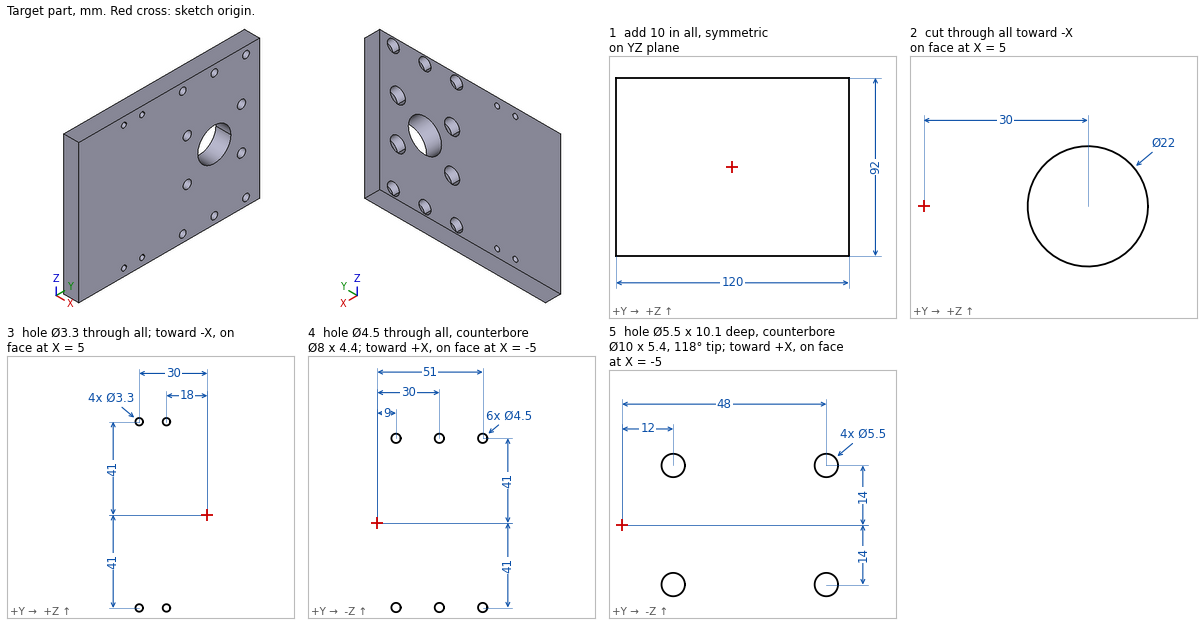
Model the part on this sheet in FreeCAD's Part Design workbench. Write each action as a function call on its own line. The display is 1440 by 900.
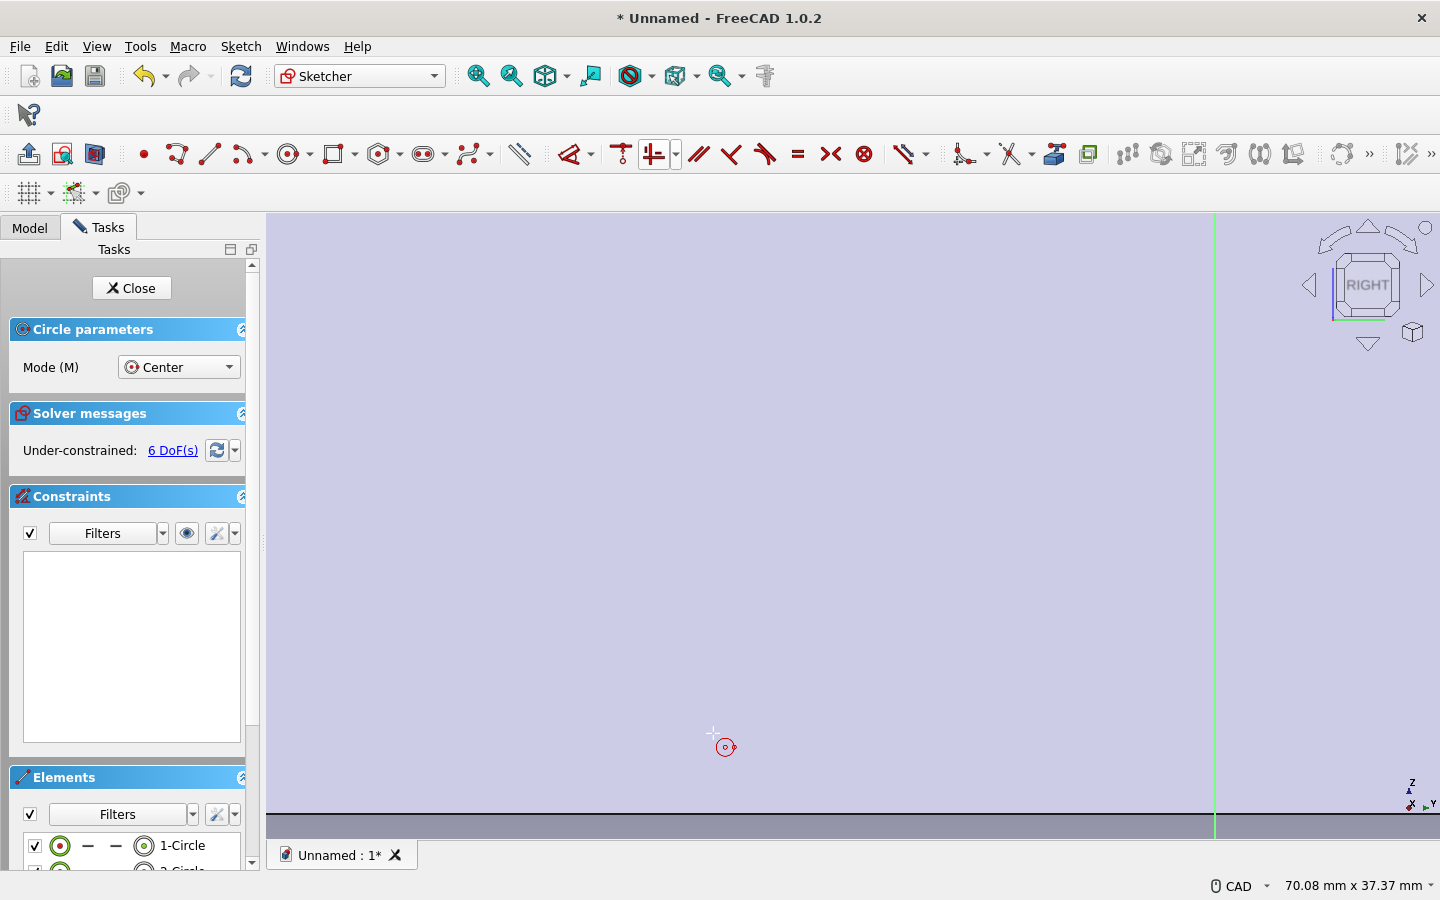
scroll(713, 734, down, 6)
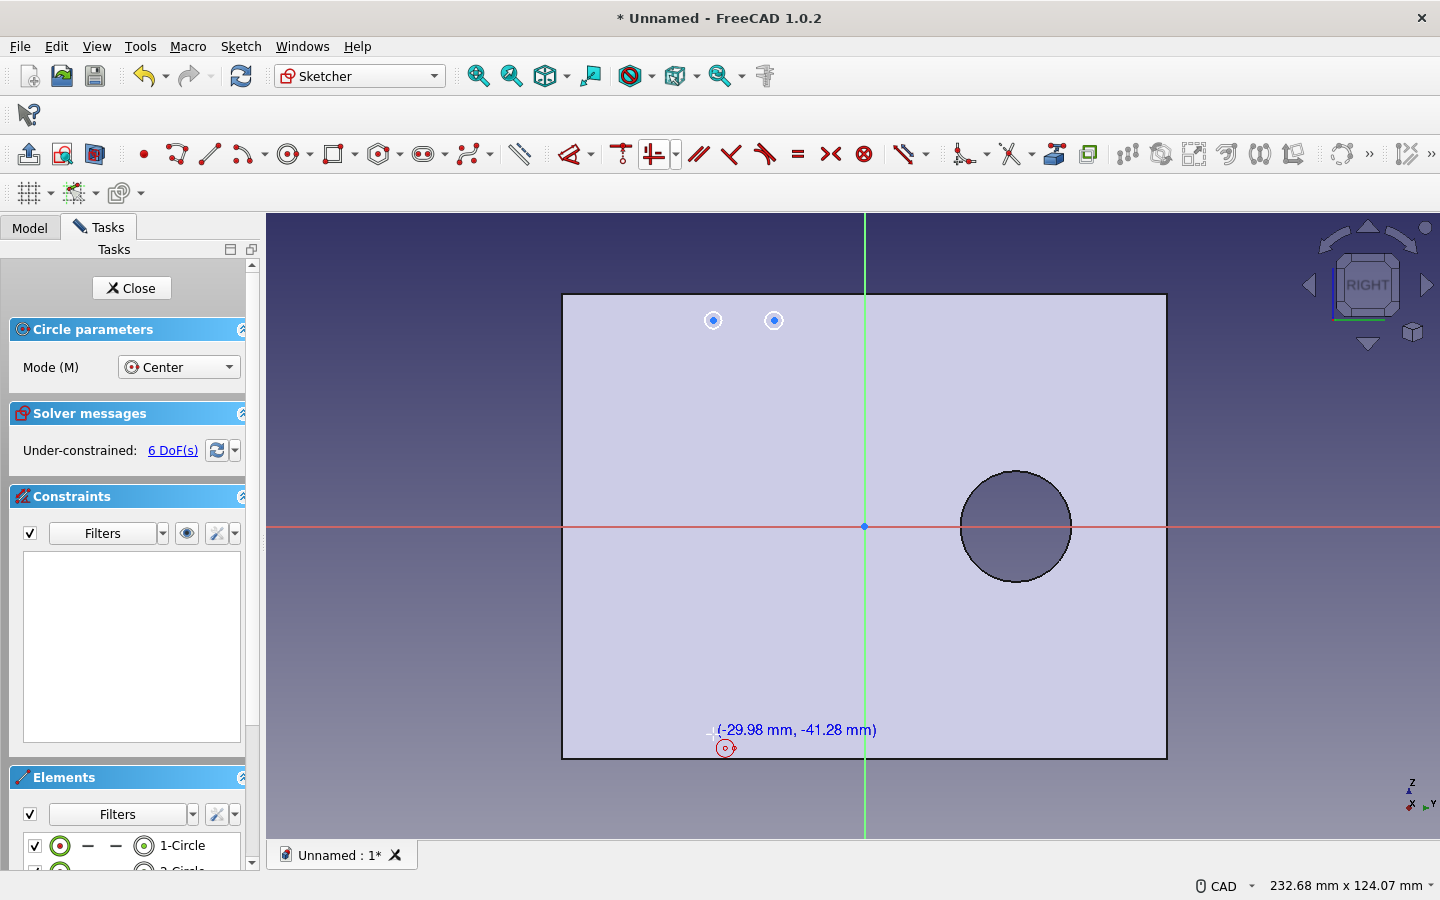
click(713, 733)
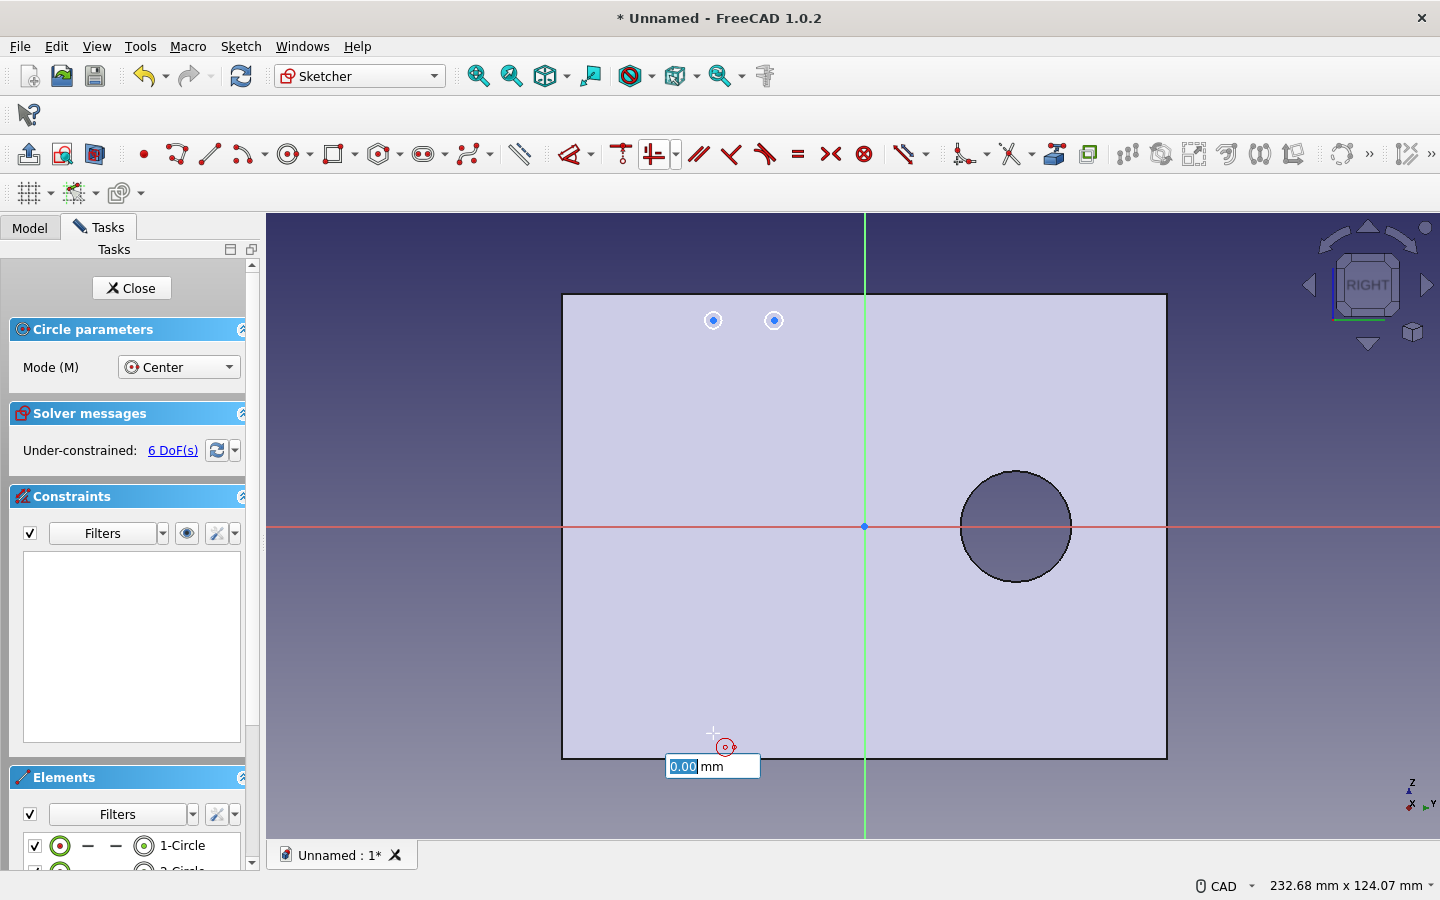
scroll(719, 728, up, 4)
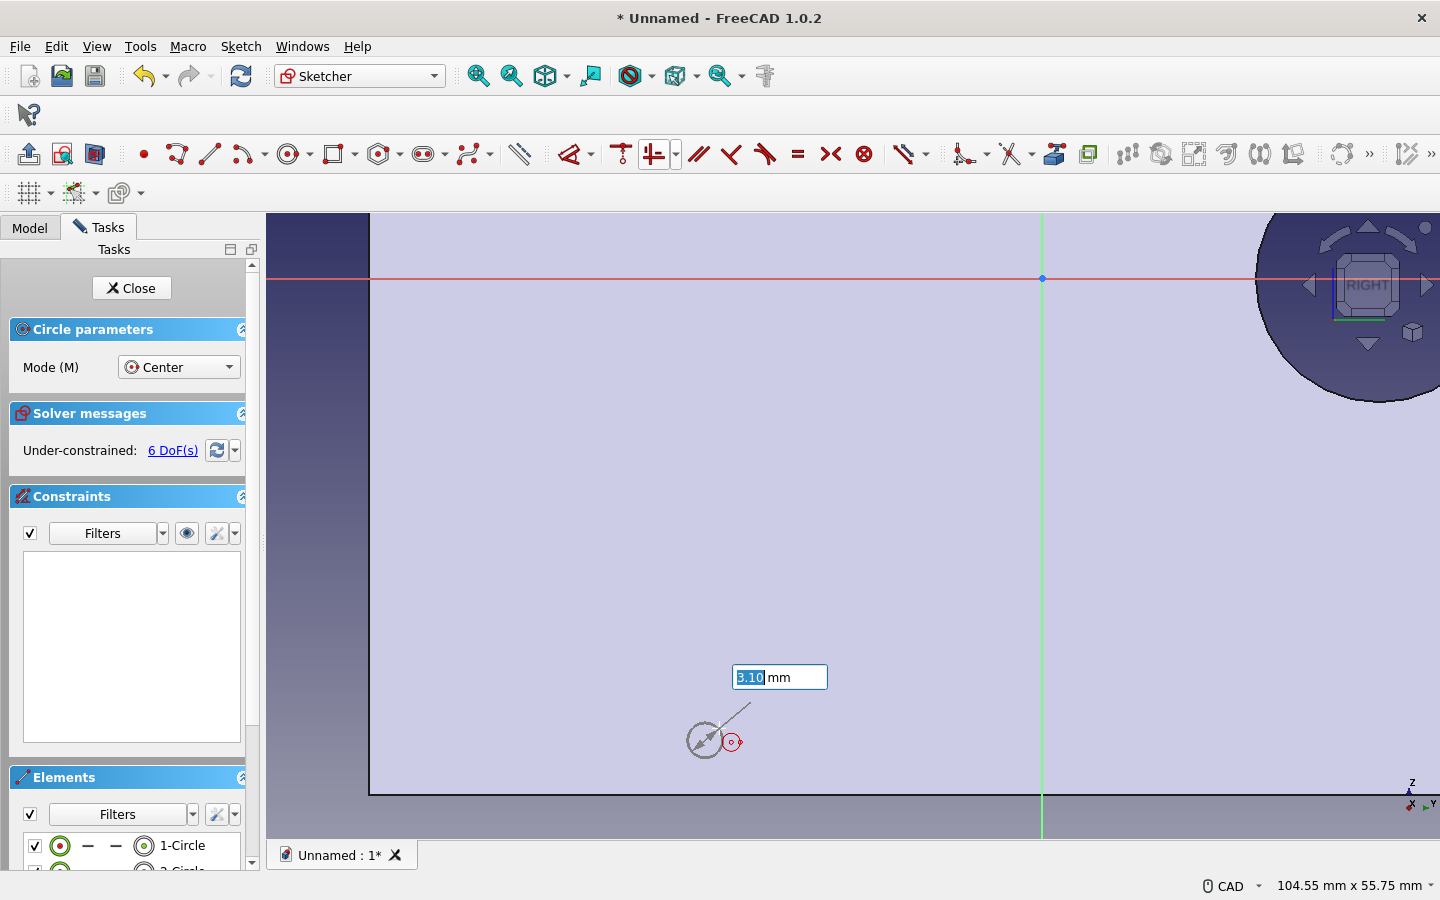
click(719, 726)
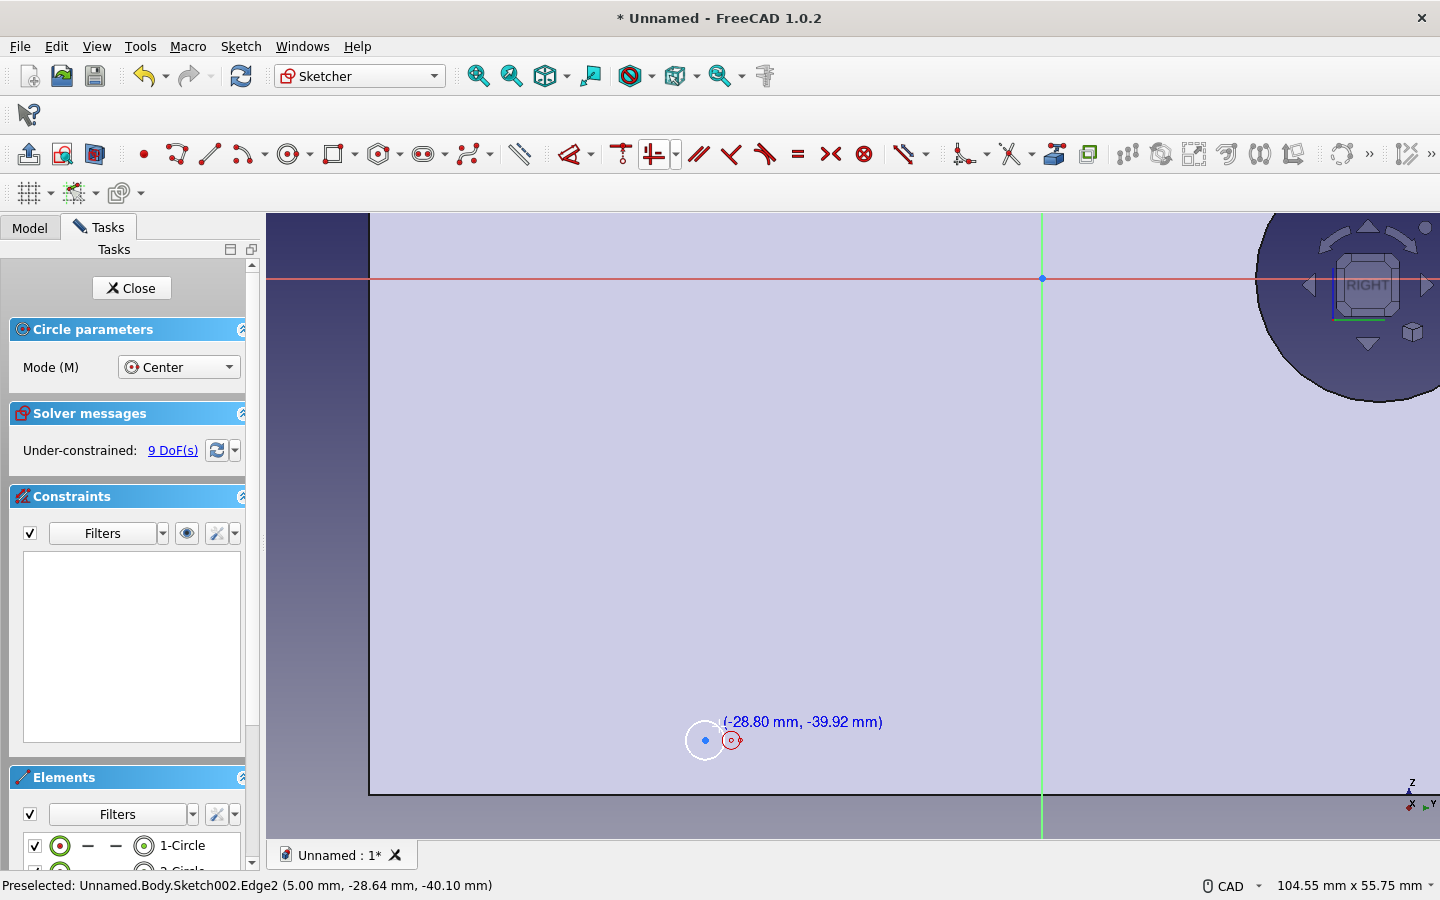
scroll(840, 739, up, 2)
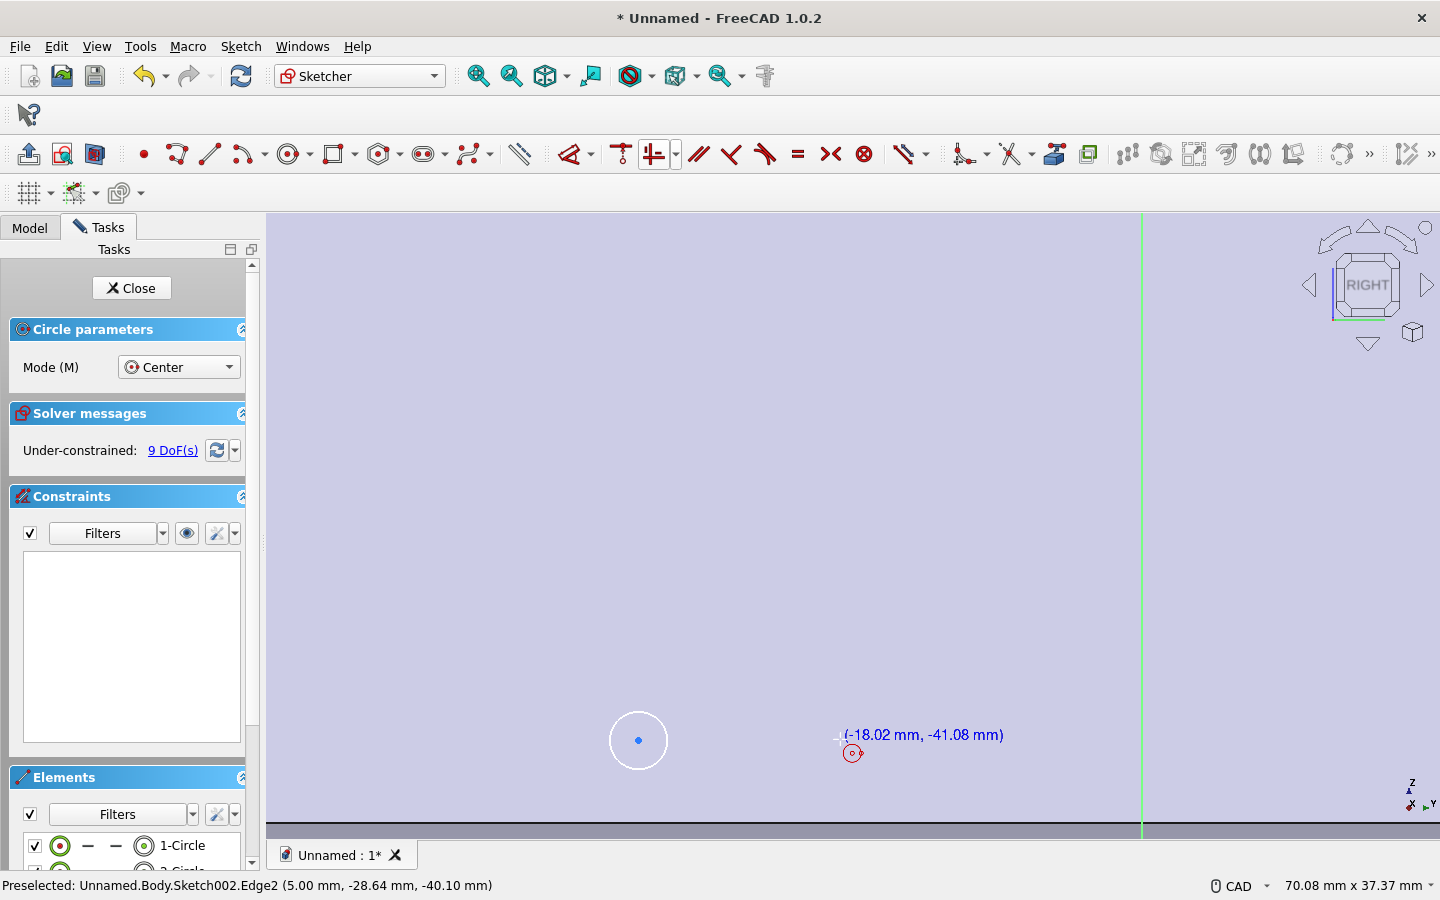
scroll(745, 730, down, 6)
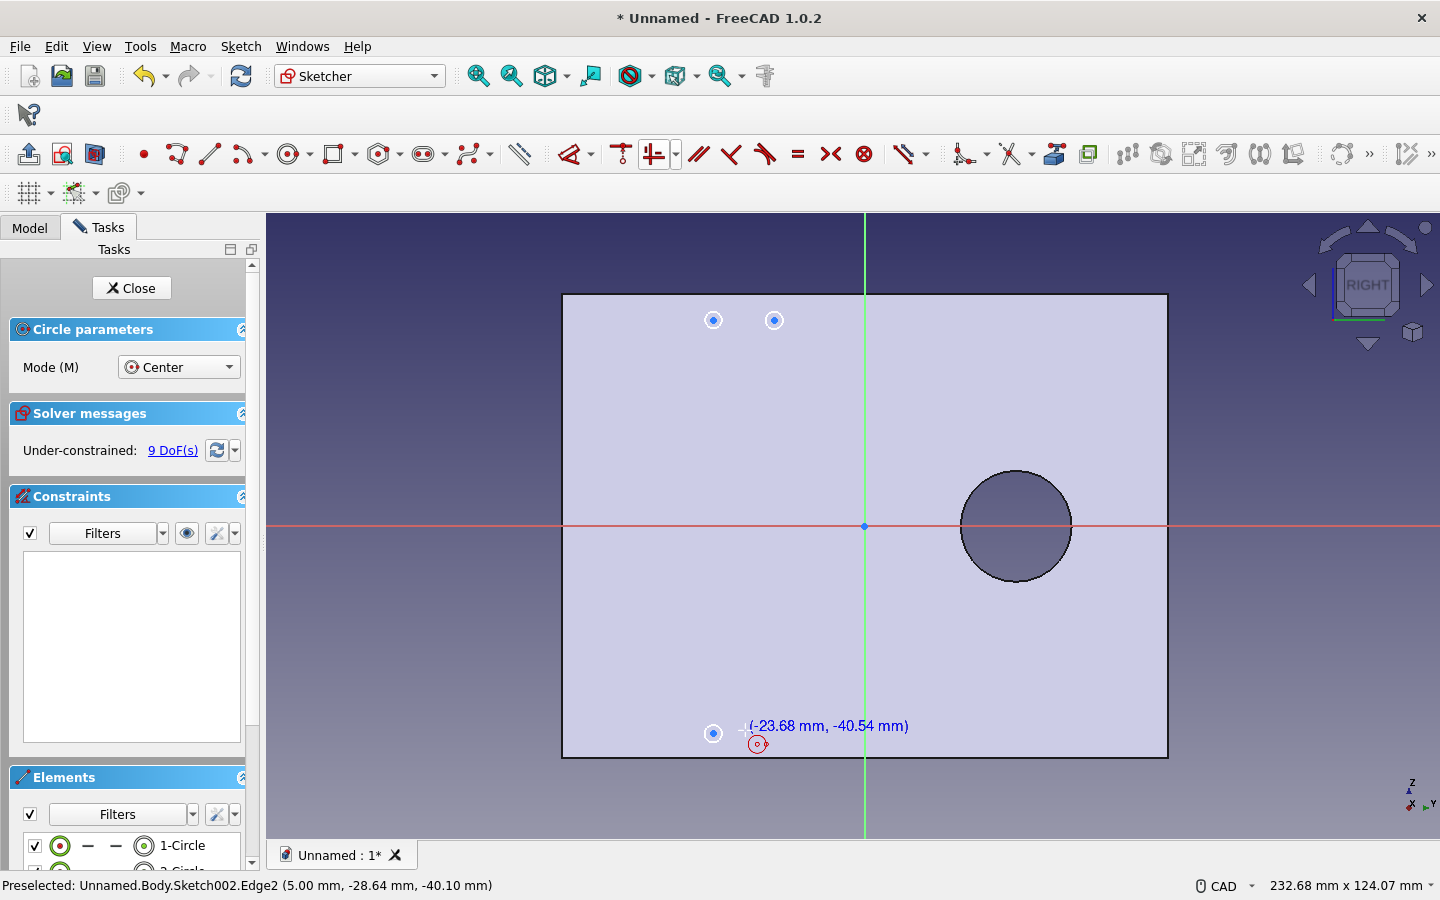
click(774, 733)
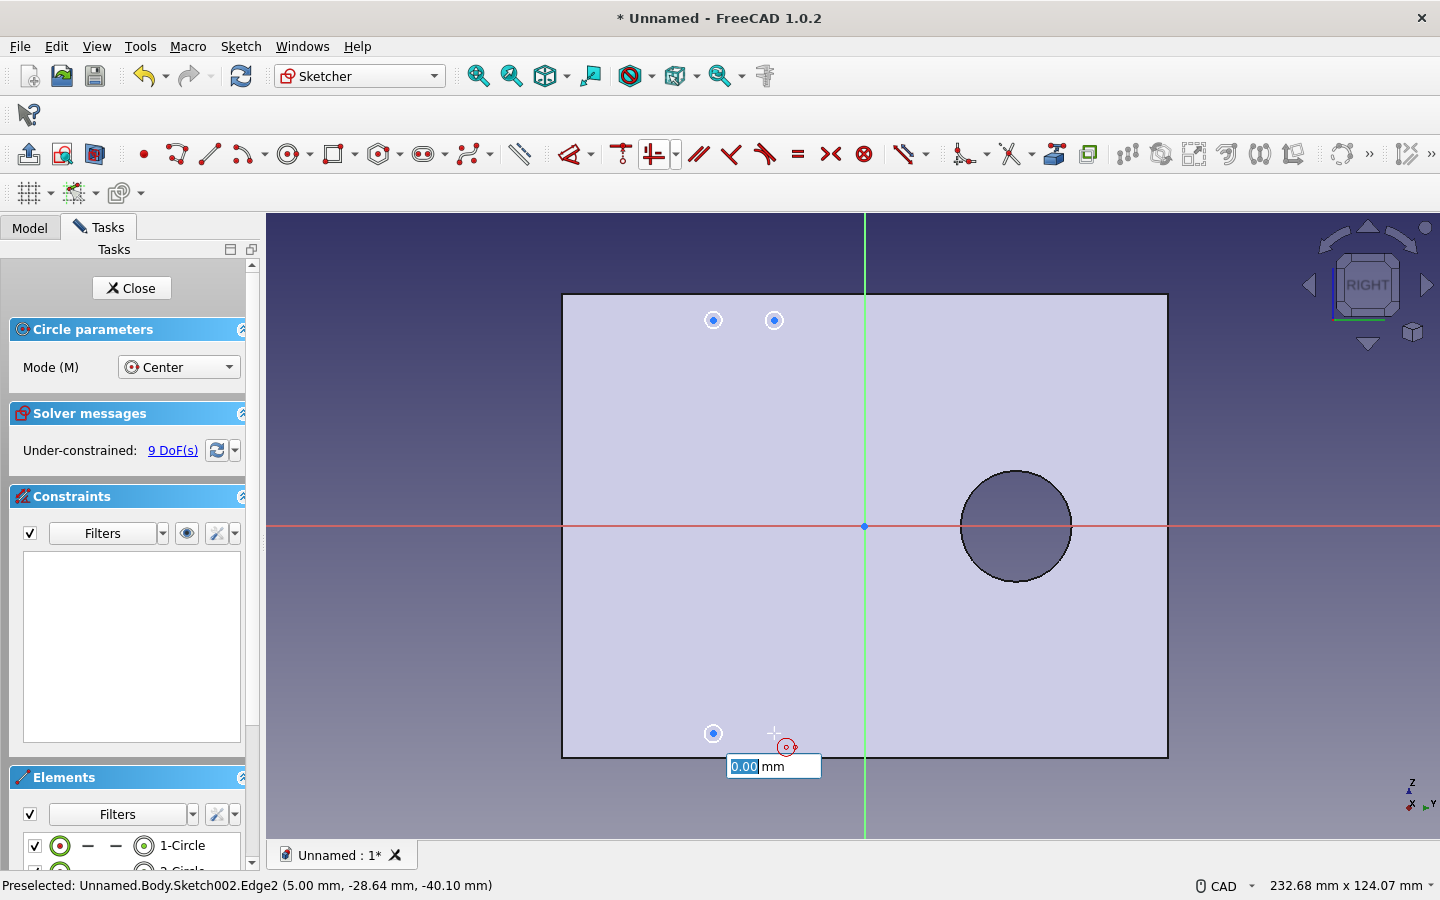
scroll(780, 727, up, 4)